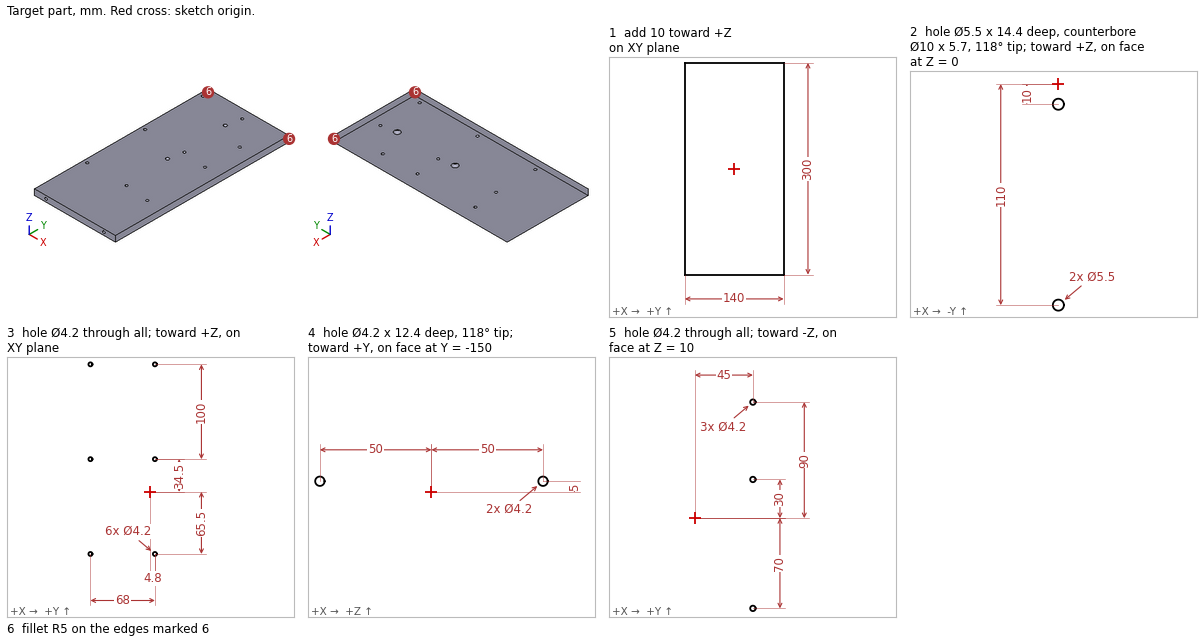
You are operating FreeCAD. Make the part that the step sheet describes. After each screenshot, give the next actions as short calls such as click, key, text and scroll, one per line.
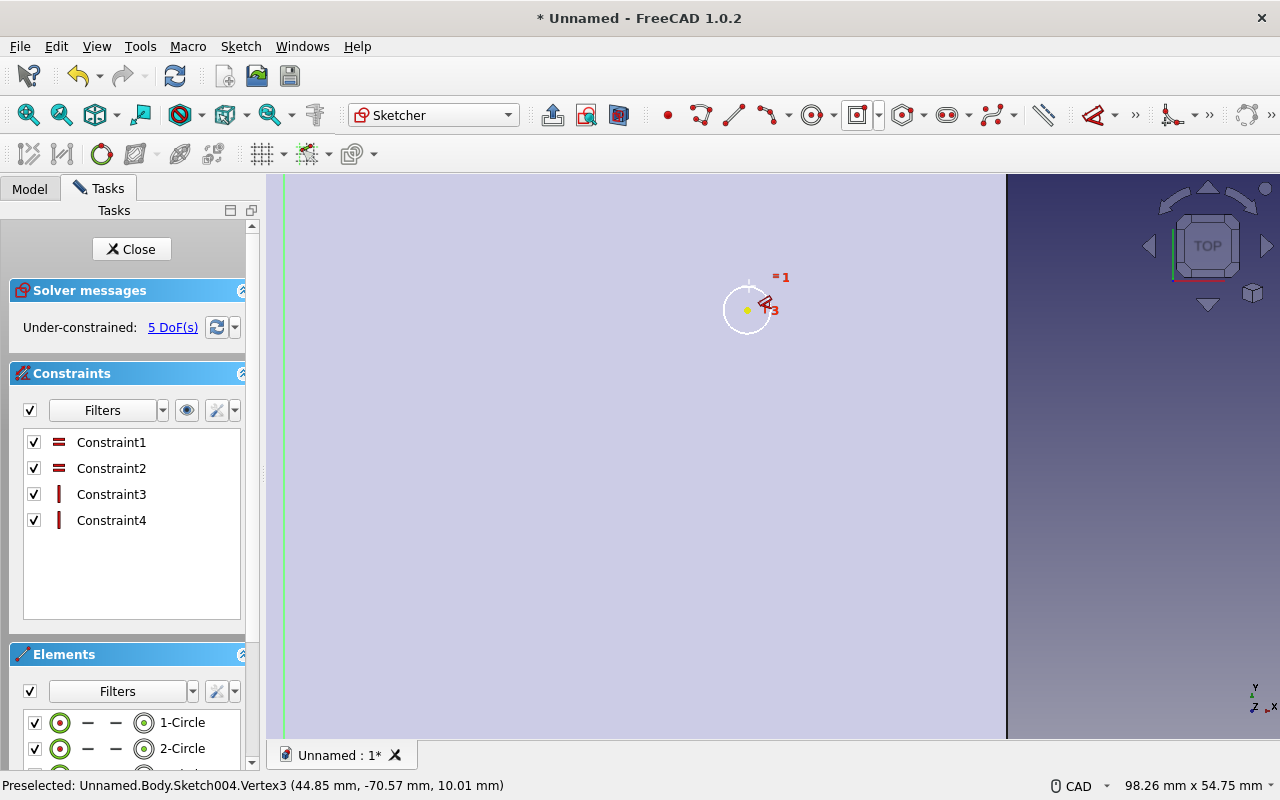
click(748, 287)
click(749, 255)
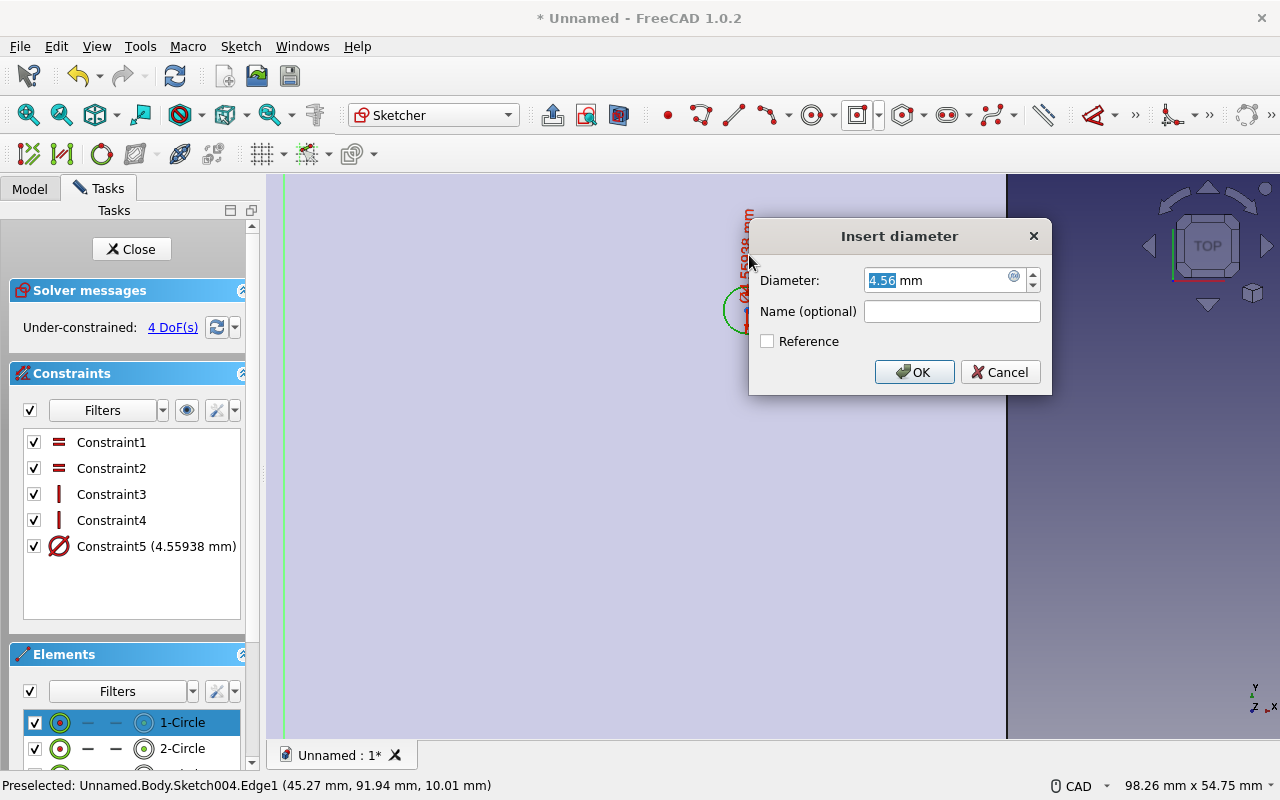
text(4.2)
key(Return)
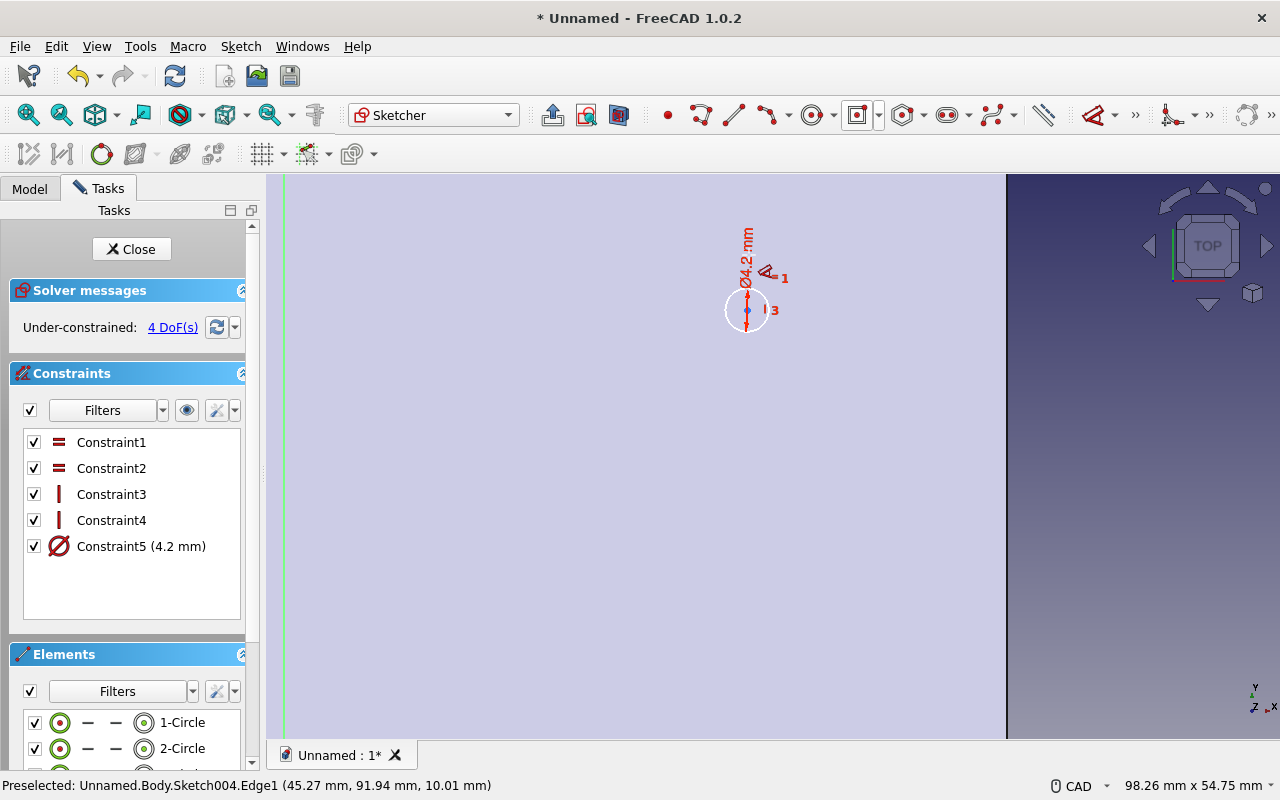
scroll(749, 285, down, 8)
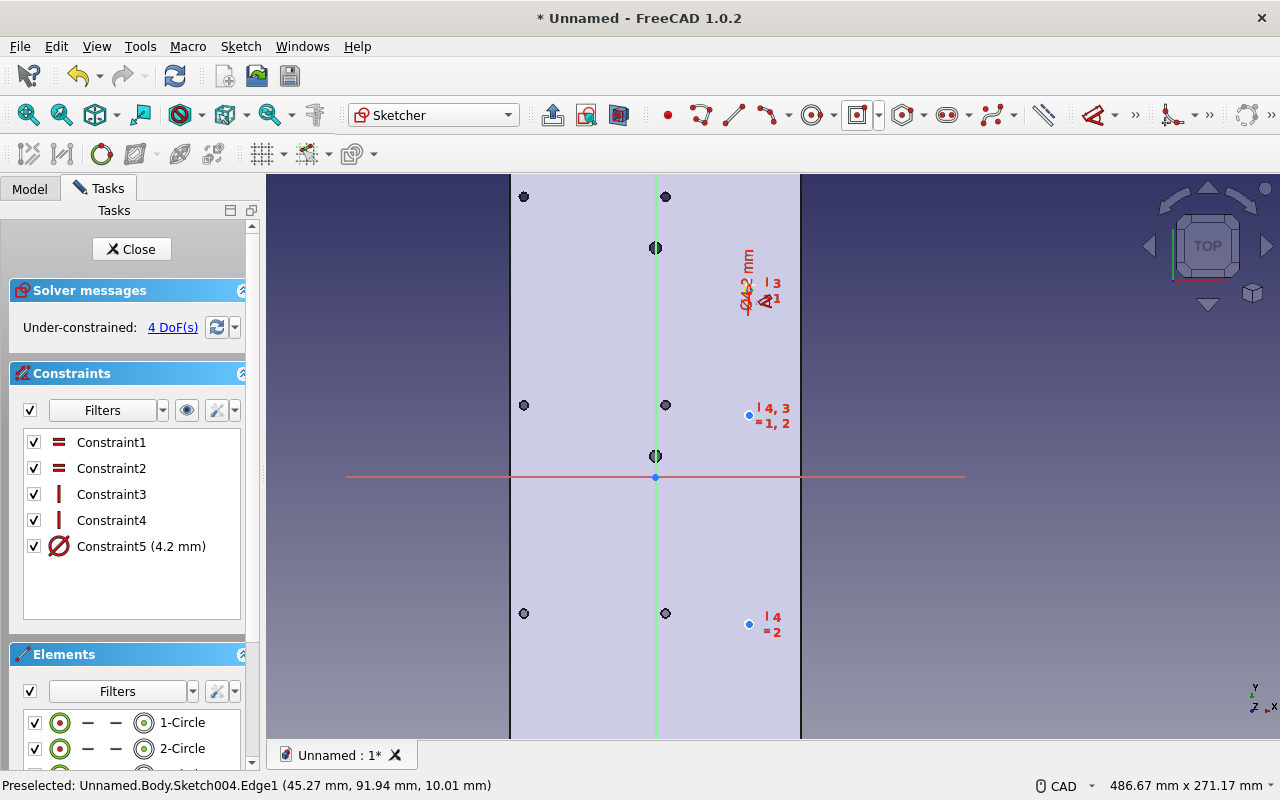
click(749, 290)
click(702, 256)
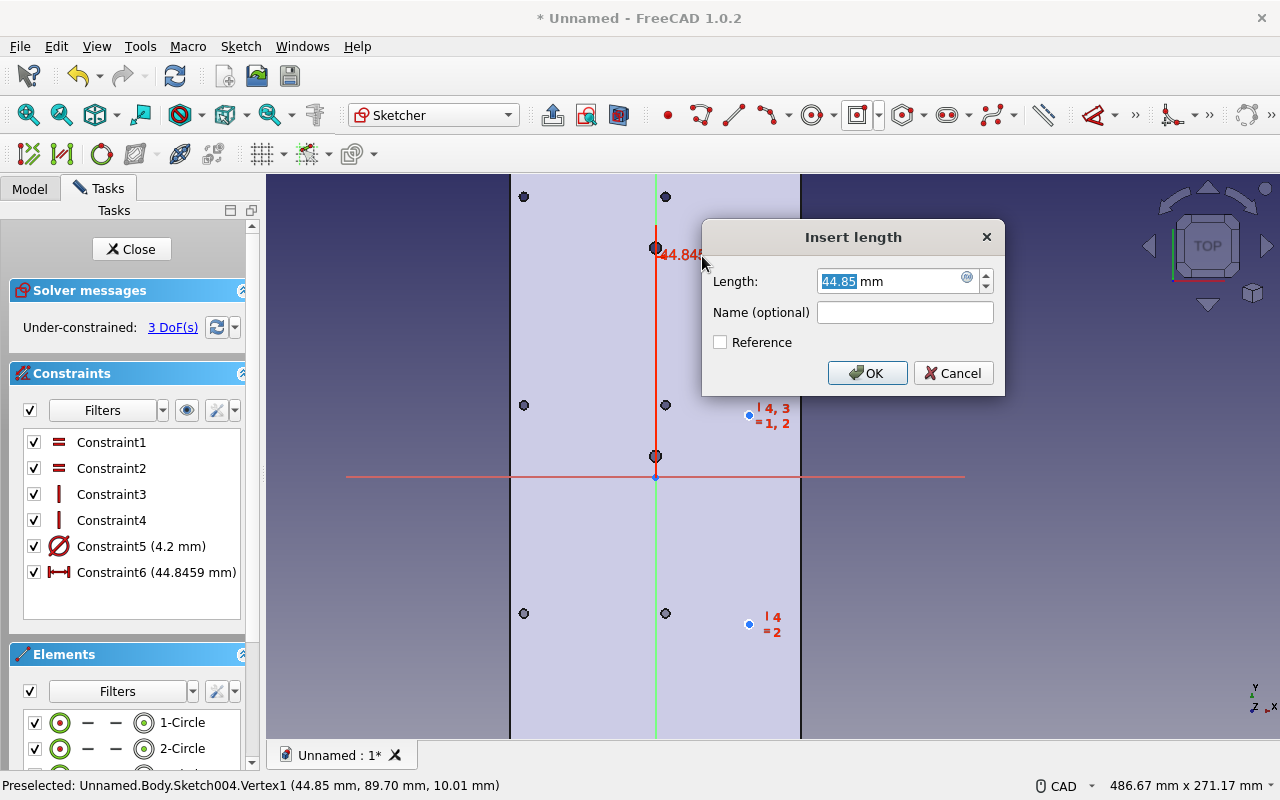
text(45)
key(Return)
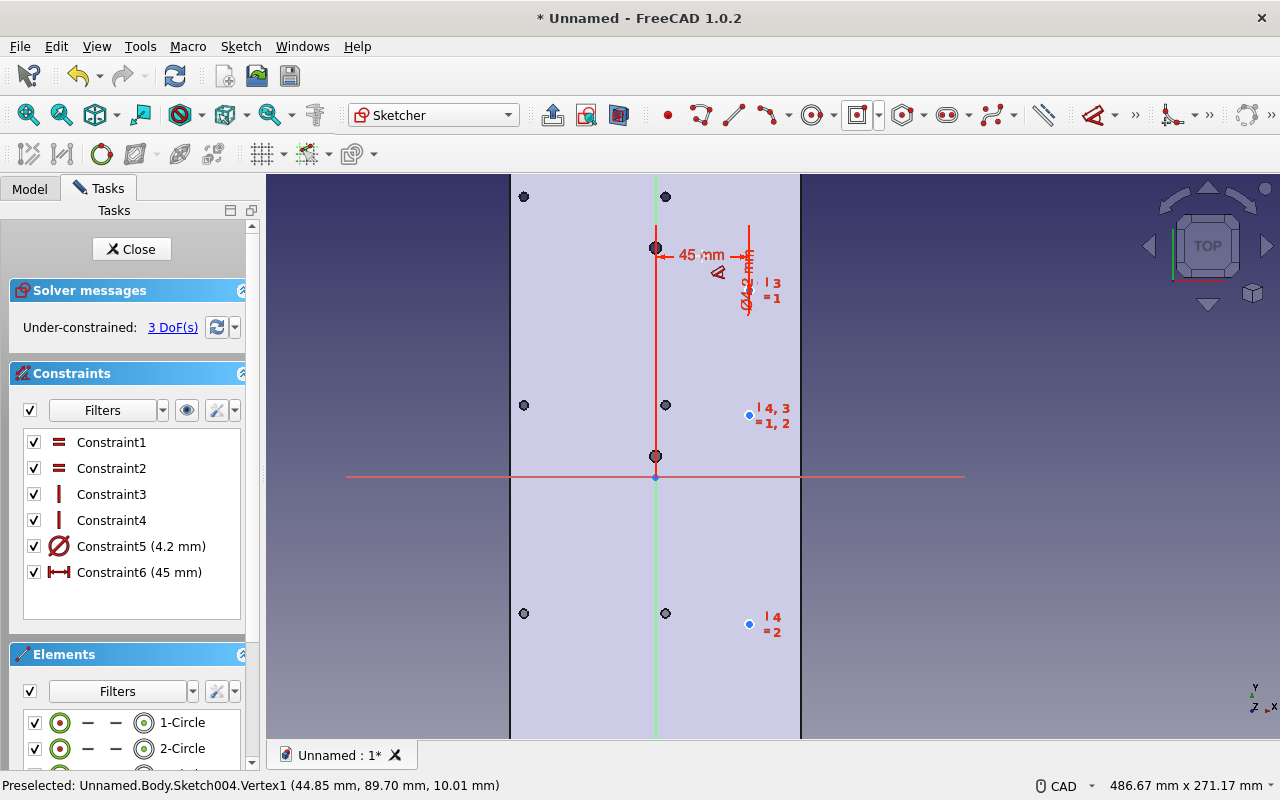
click(749, 290)
click(622, 384)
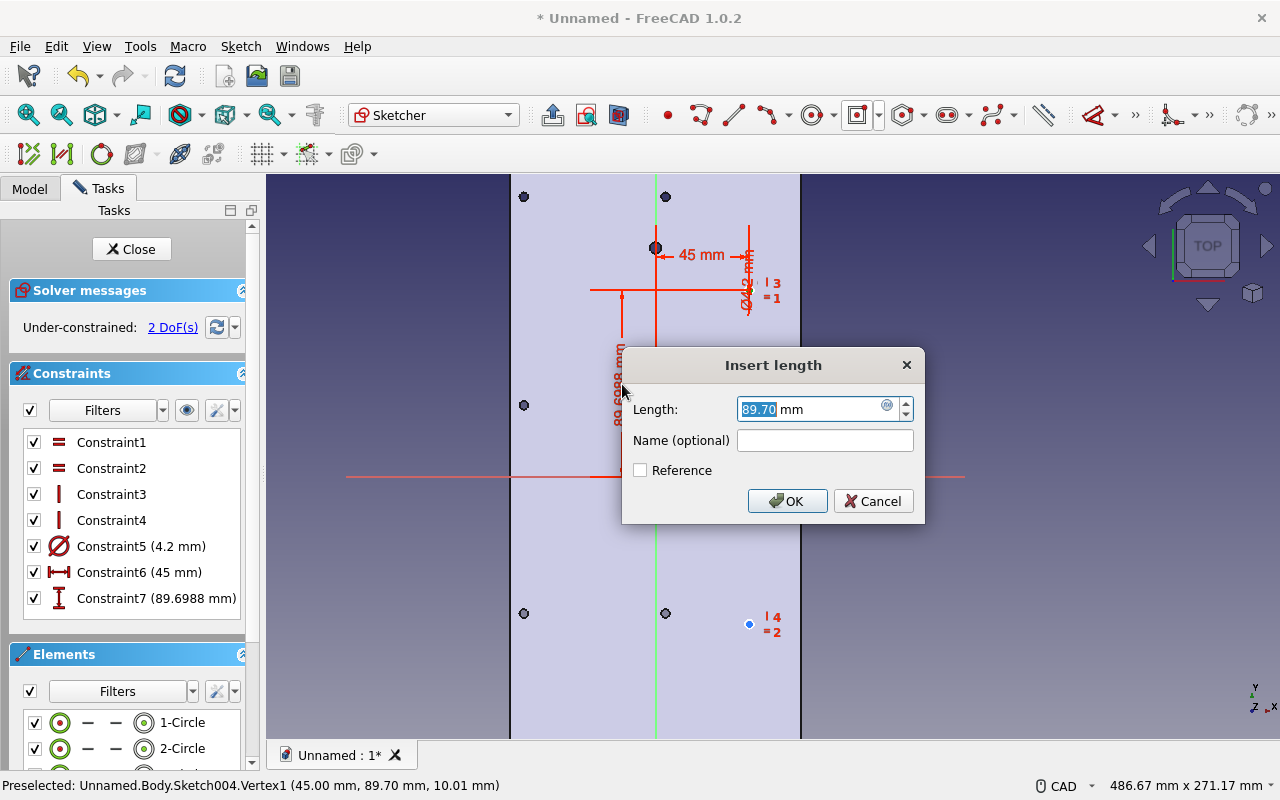
text(90)
key(Return)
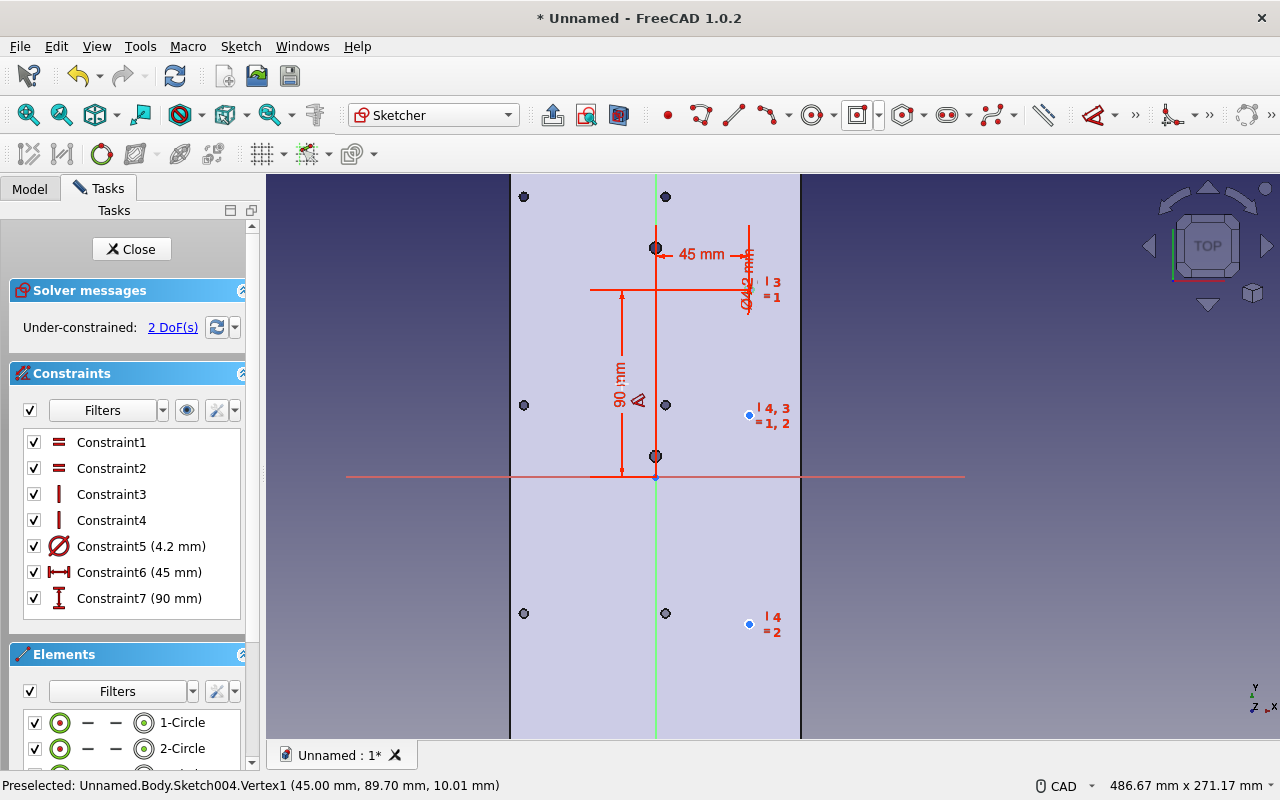
click(749, 415)
click(622, 446)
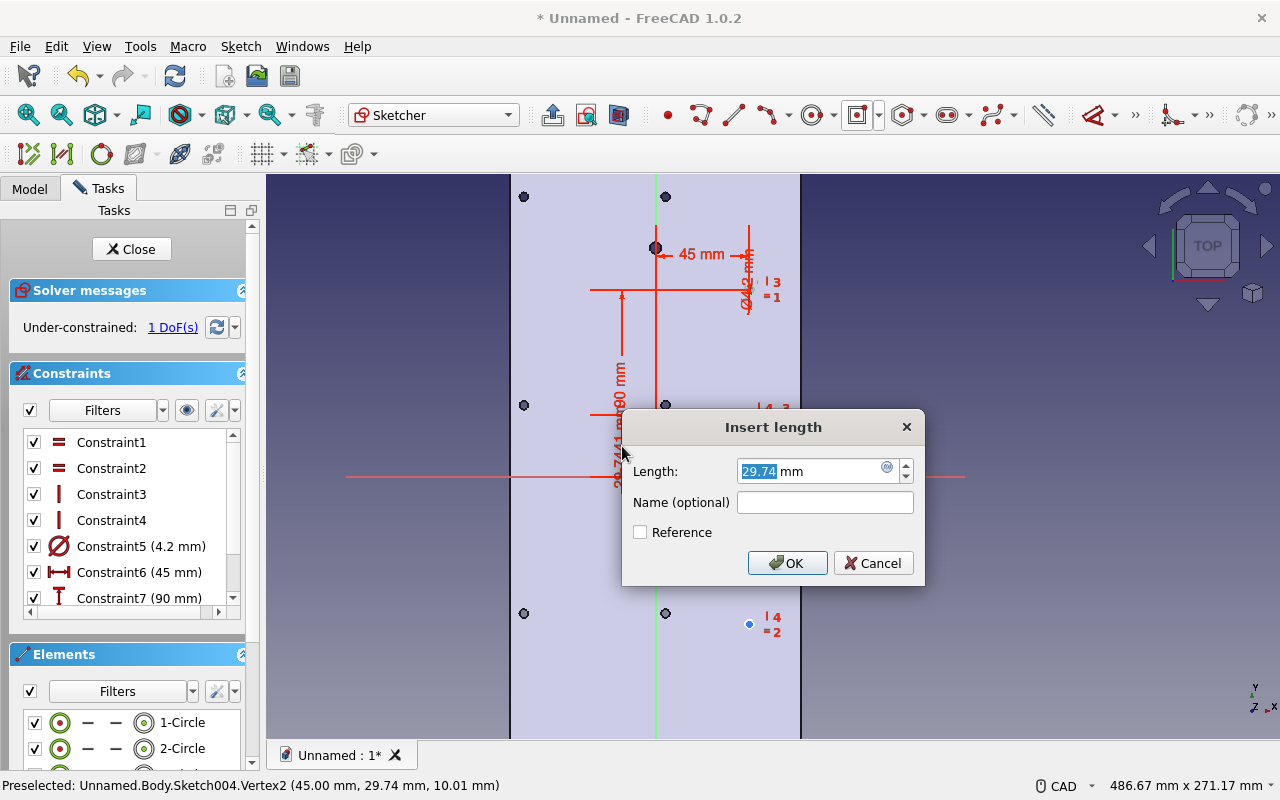
text(30)
key(Return)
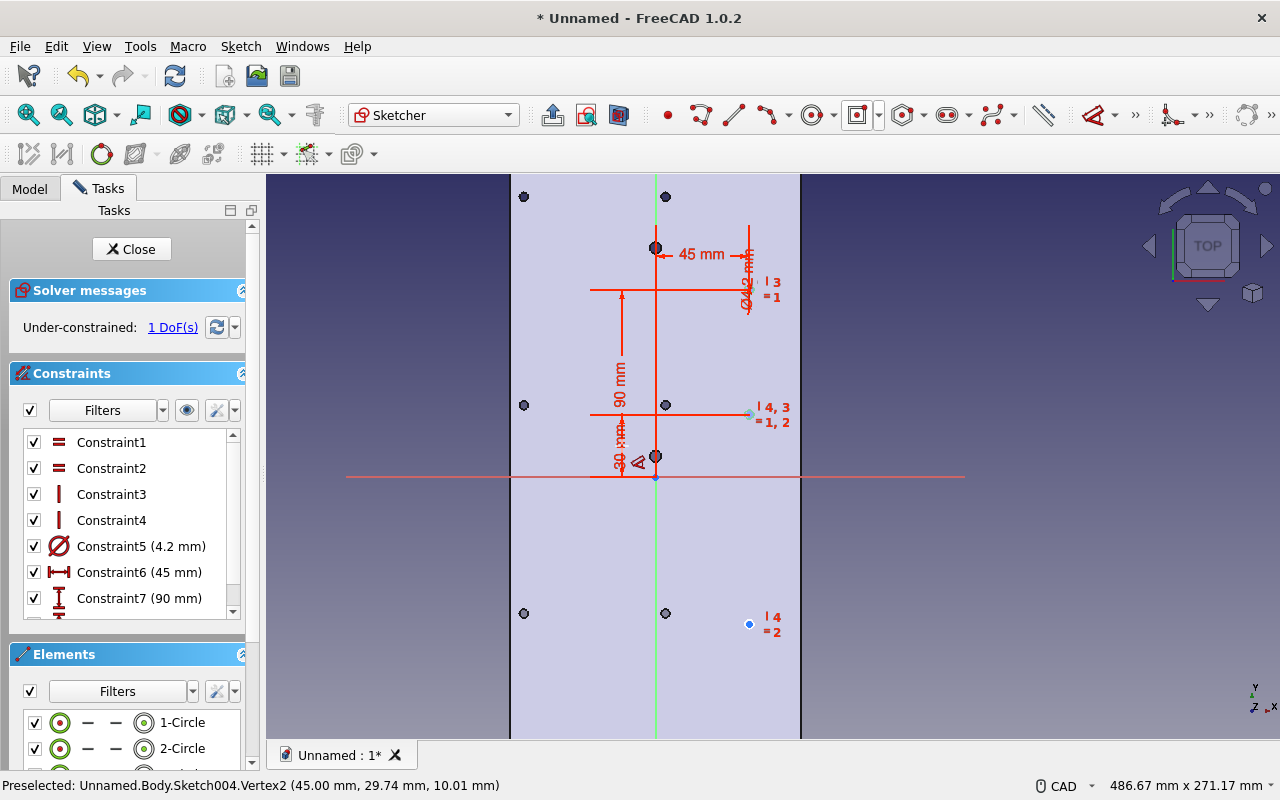
click(749, 624)
click(622, 551)